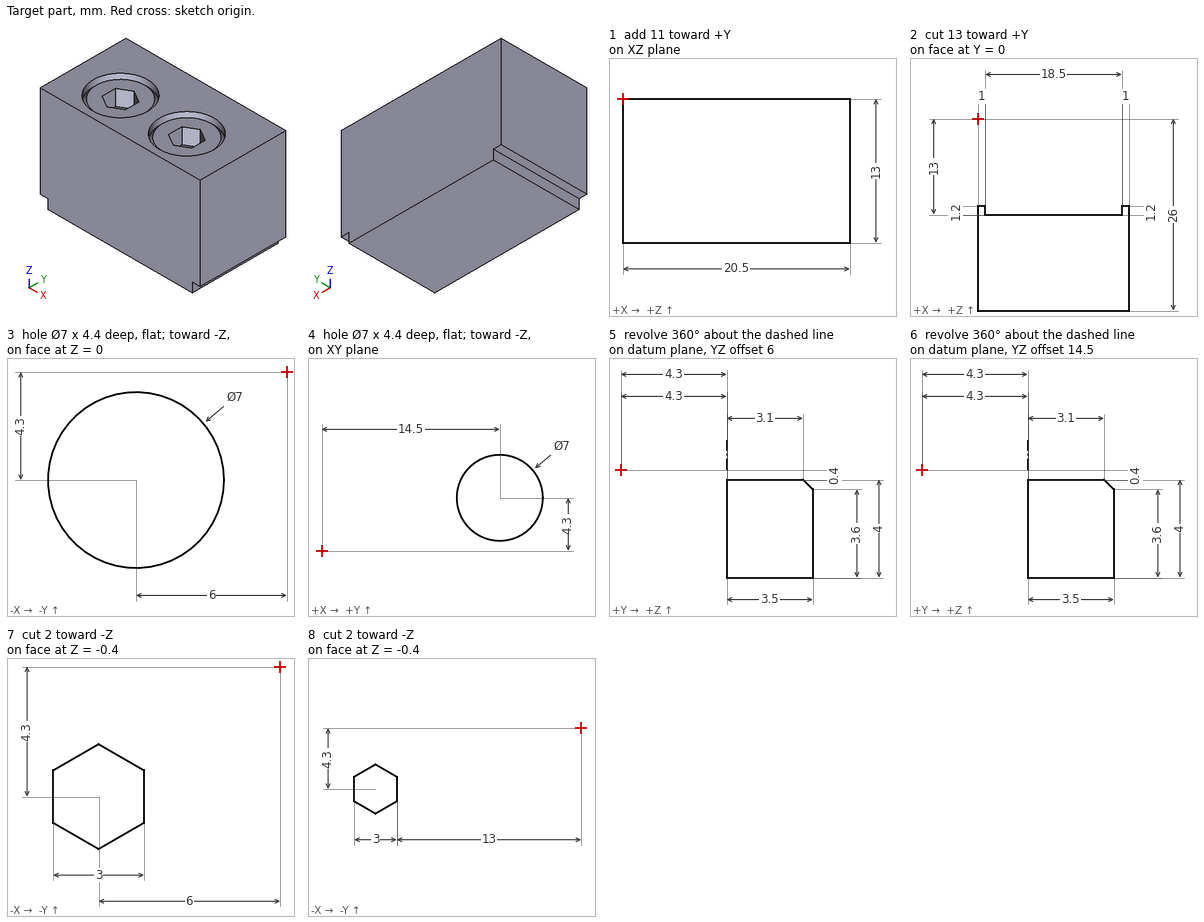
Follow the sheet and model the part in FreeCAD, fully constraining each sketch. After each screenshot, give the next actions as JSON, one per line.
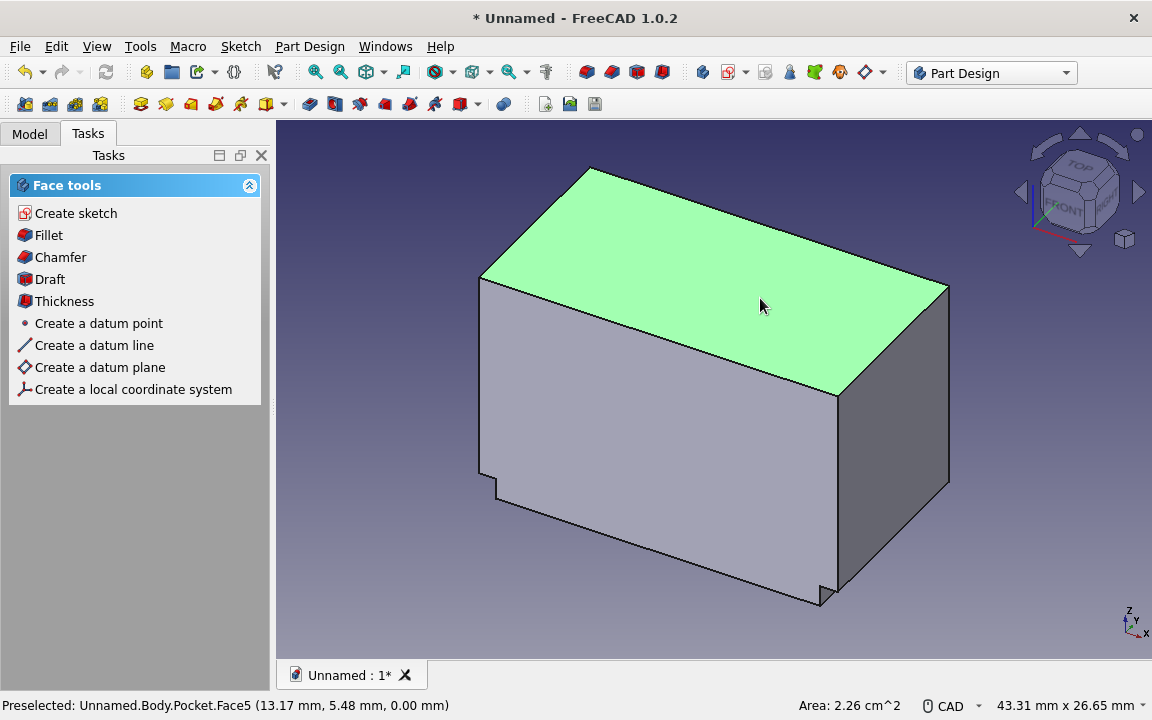
{"action": "left_click", "coordinate": [728, 72]}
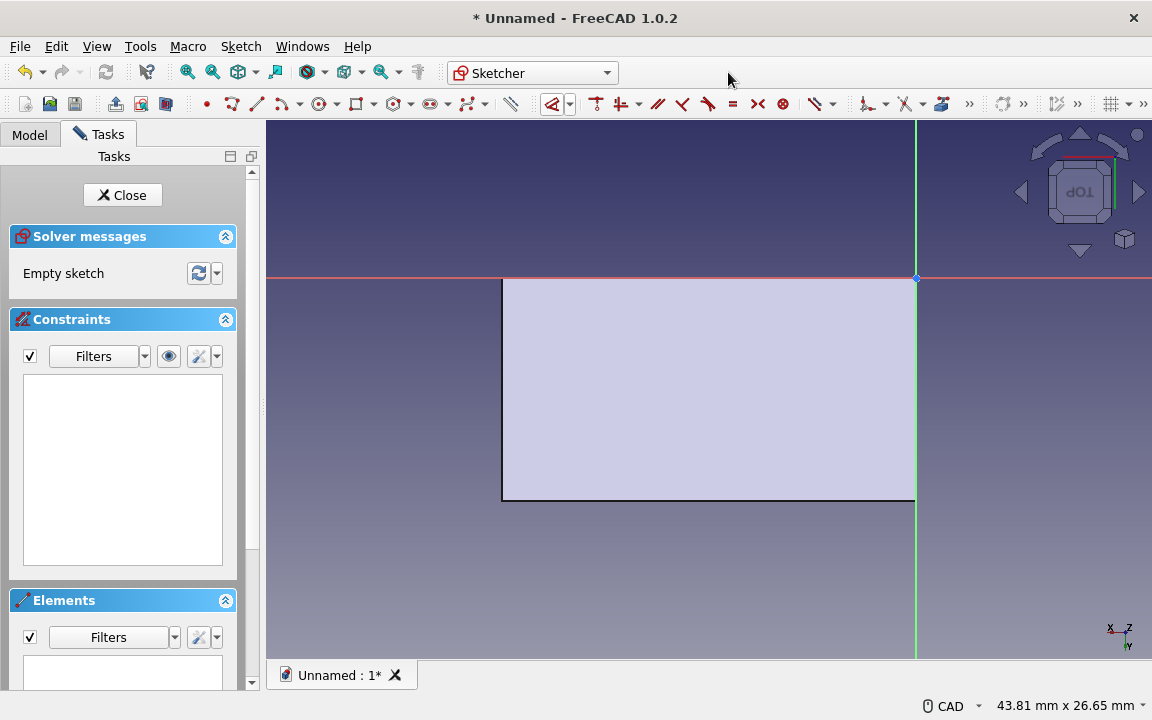
{"action": "scroll", "coordinate": [967, 331], "scroll_direction": "up", "scroll_amount": 4}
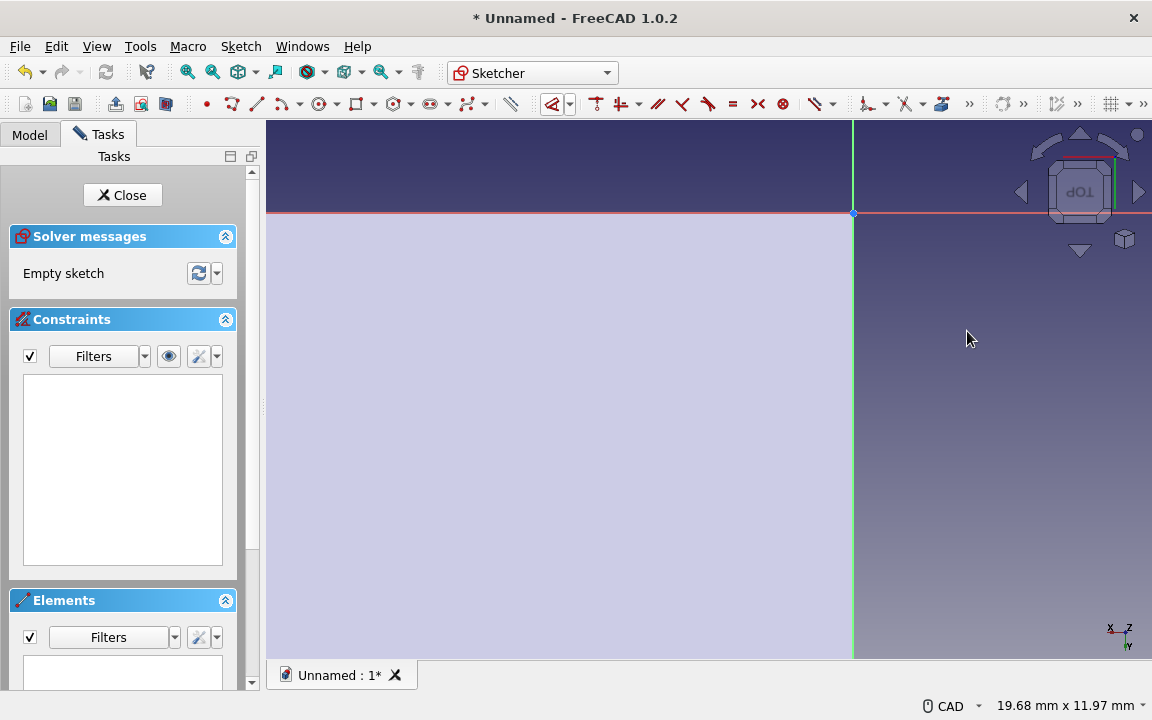
{"action": "key", "text": "g c"}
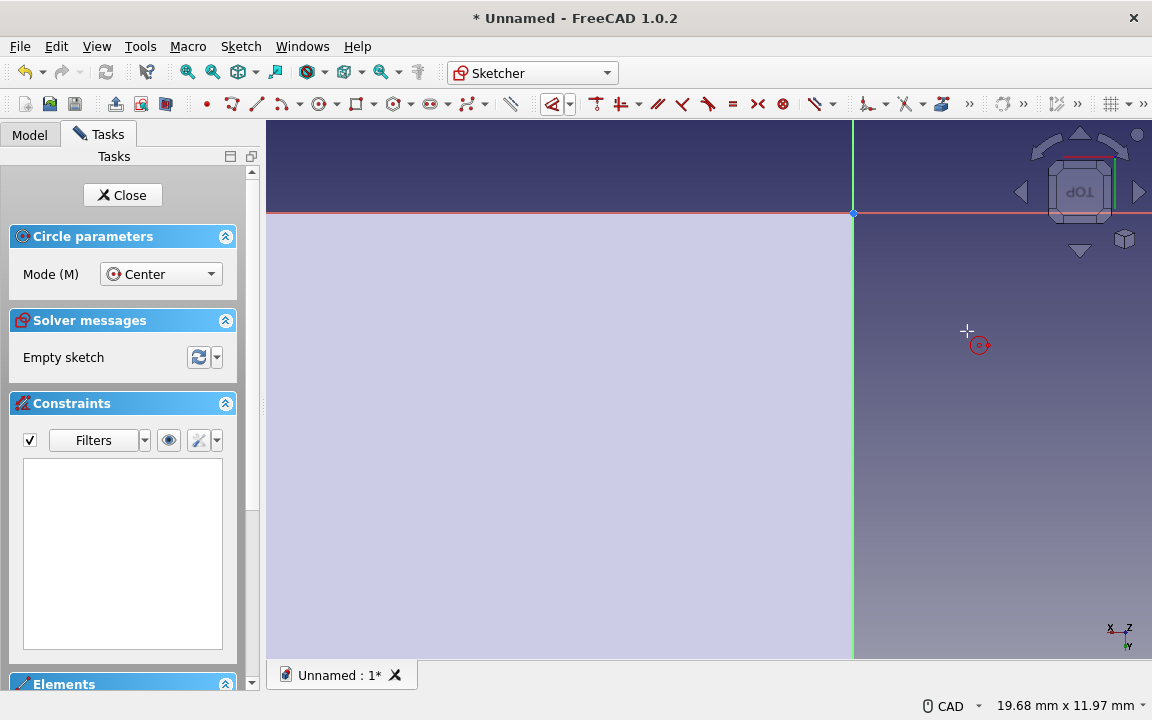
{"action": "left_click", "coordinate": [583, 407]}
{"action": "mouse_move", "coordinate": [695, 295]}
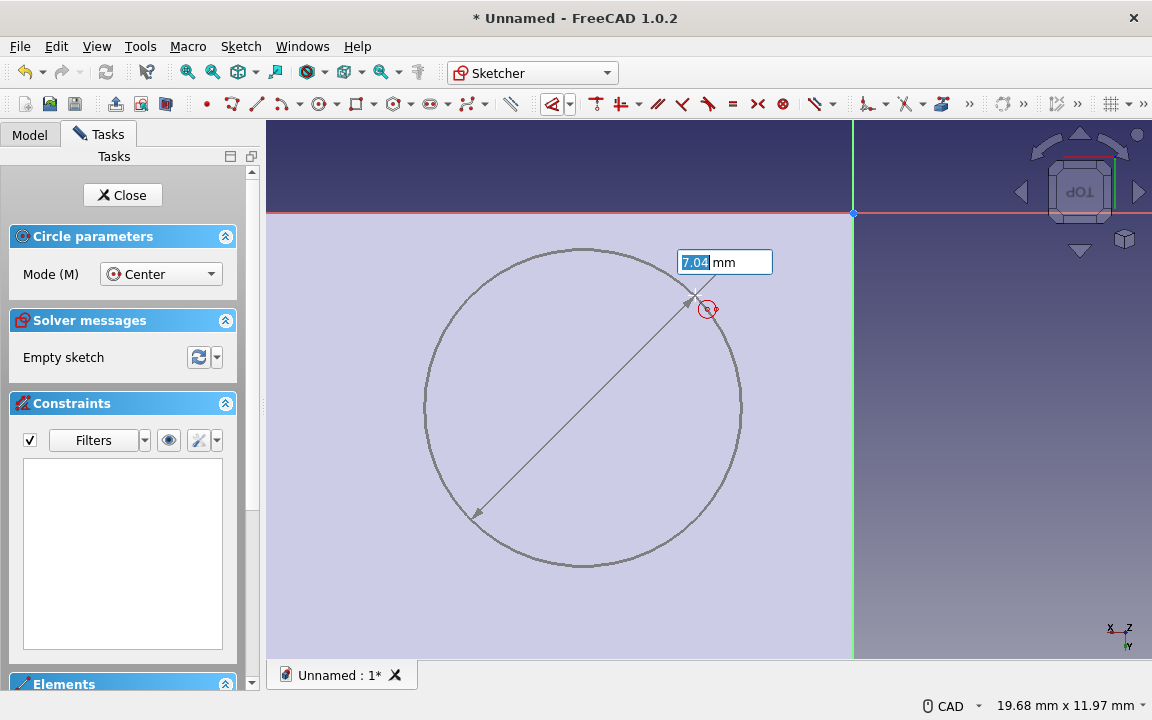
{"action": "type", "text": "7"}
{"action": "key", "text": "Return"}
{"action": "key", "text": "Escape"}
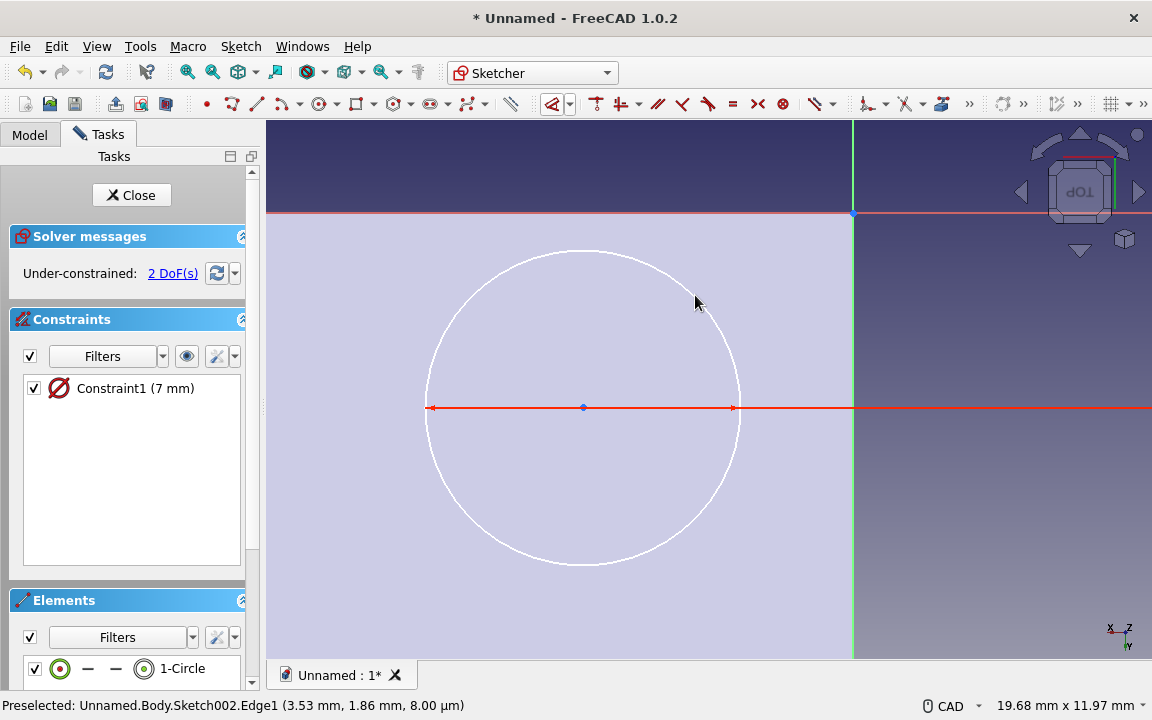
{"action": "left_click", "coordinate": [583, 408]}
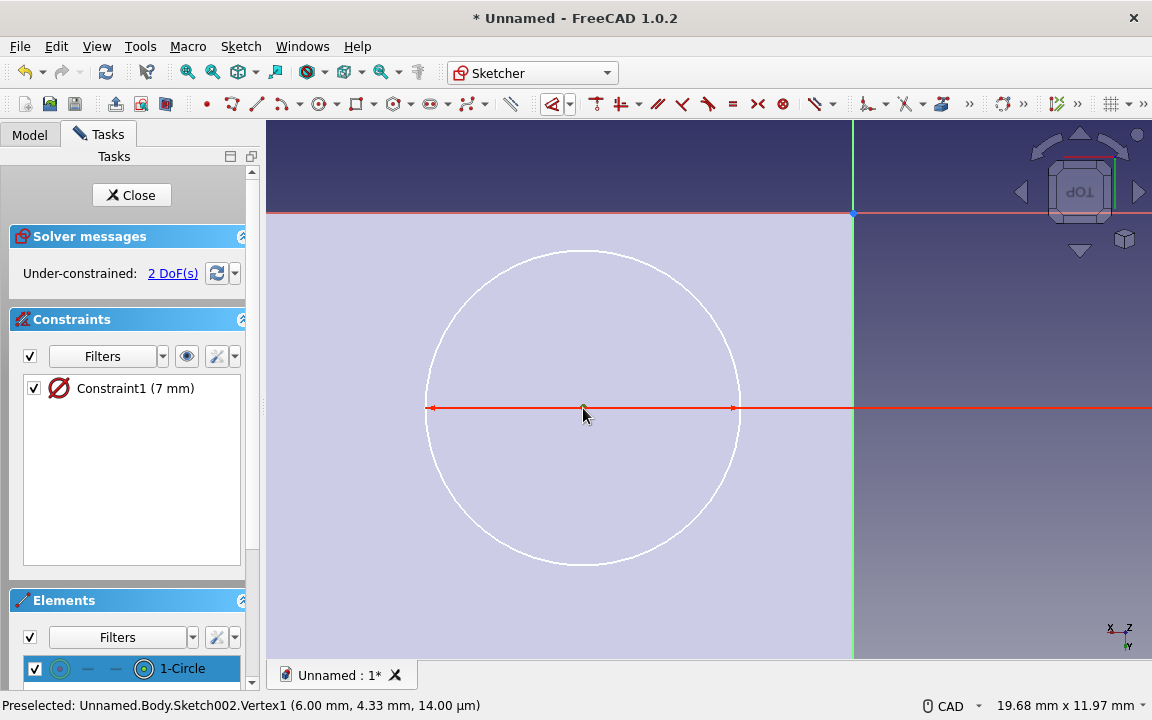
{"action": "left_click", "coordinate": [570, 104]}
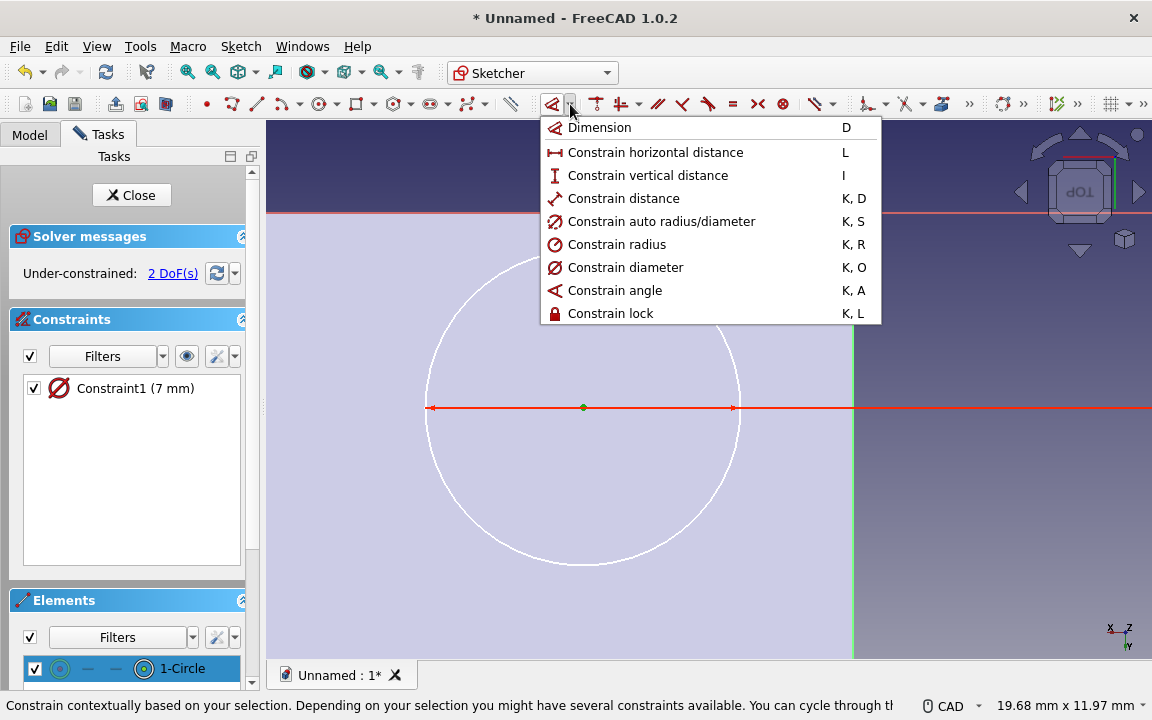
{"action": "left_click", "coordinate": [711, 152]}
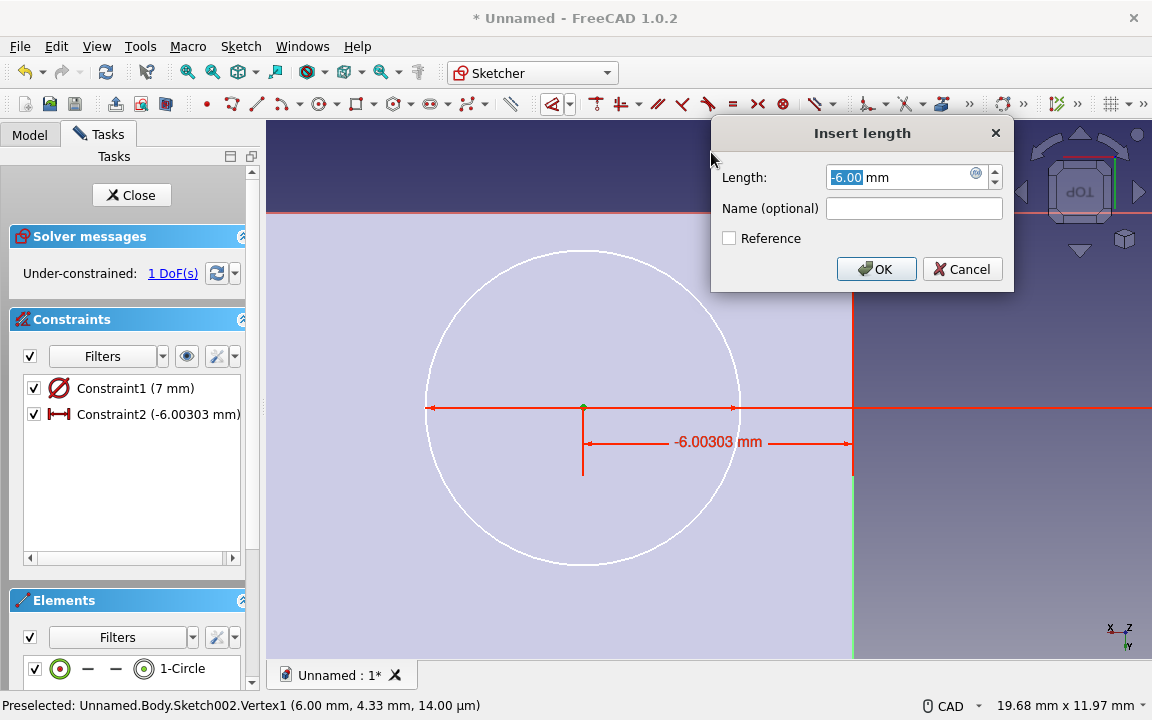
{"action": "type", "text": "-6"}
{"action": "key", "text": "Return"}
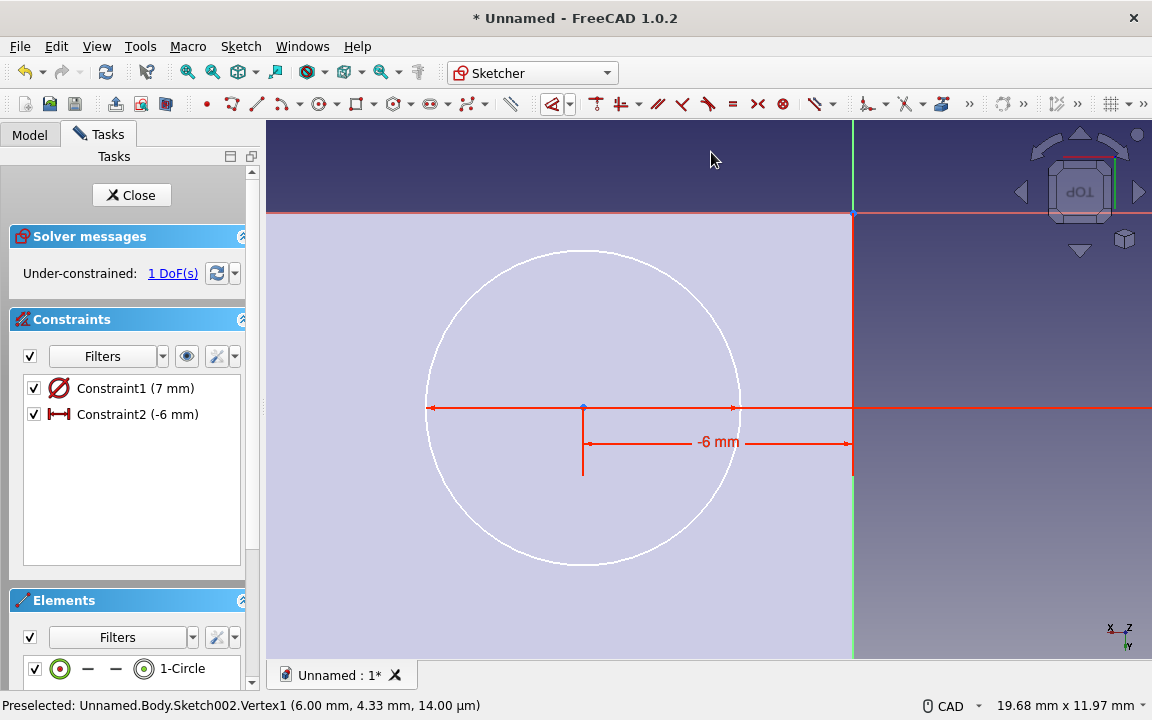
{"action": "left_click", "coordinate": [583, 408]}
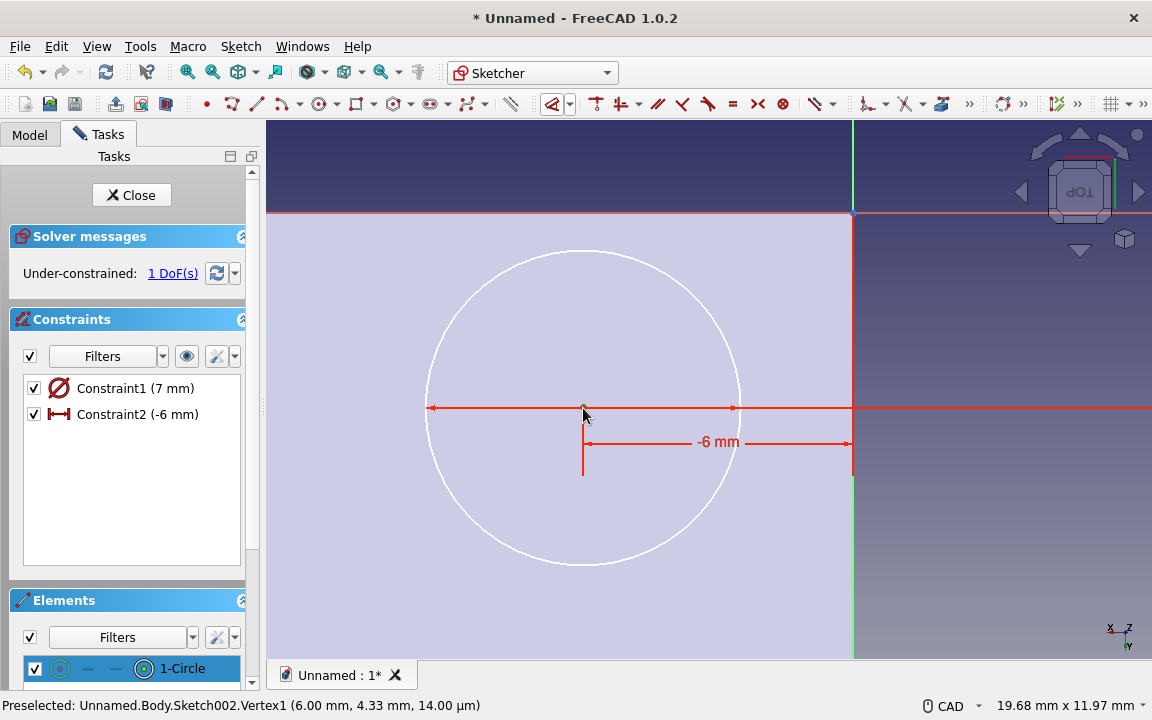
{"action": "key", "text": "i"}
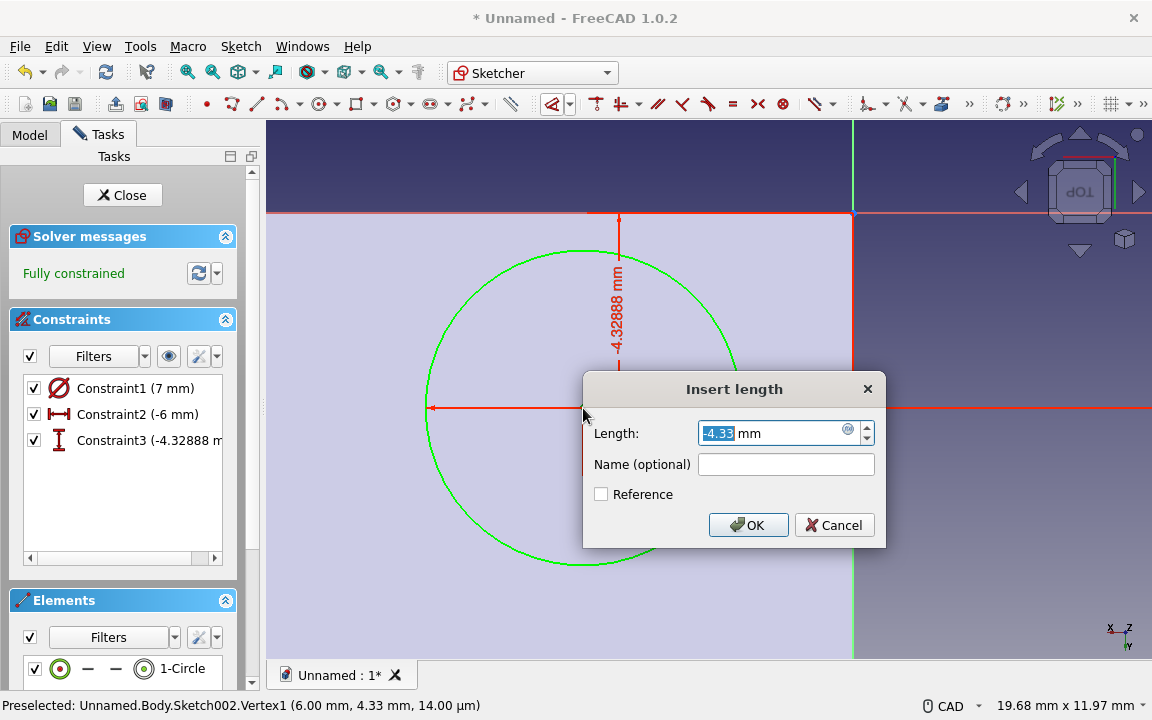
{"action": "type", "text": "-4.3"}
{"action": "key", "text": "Return"}